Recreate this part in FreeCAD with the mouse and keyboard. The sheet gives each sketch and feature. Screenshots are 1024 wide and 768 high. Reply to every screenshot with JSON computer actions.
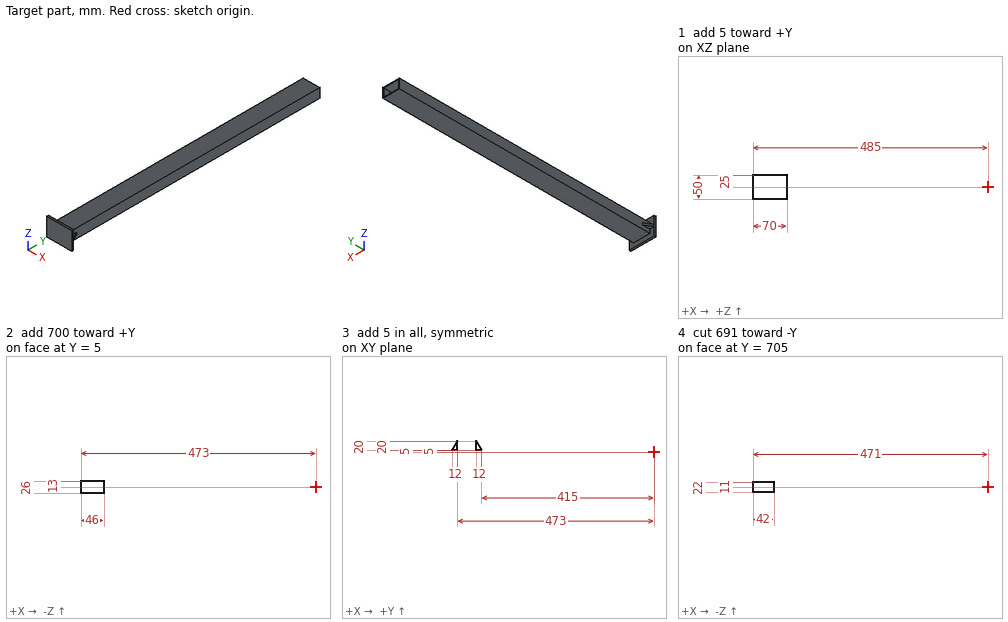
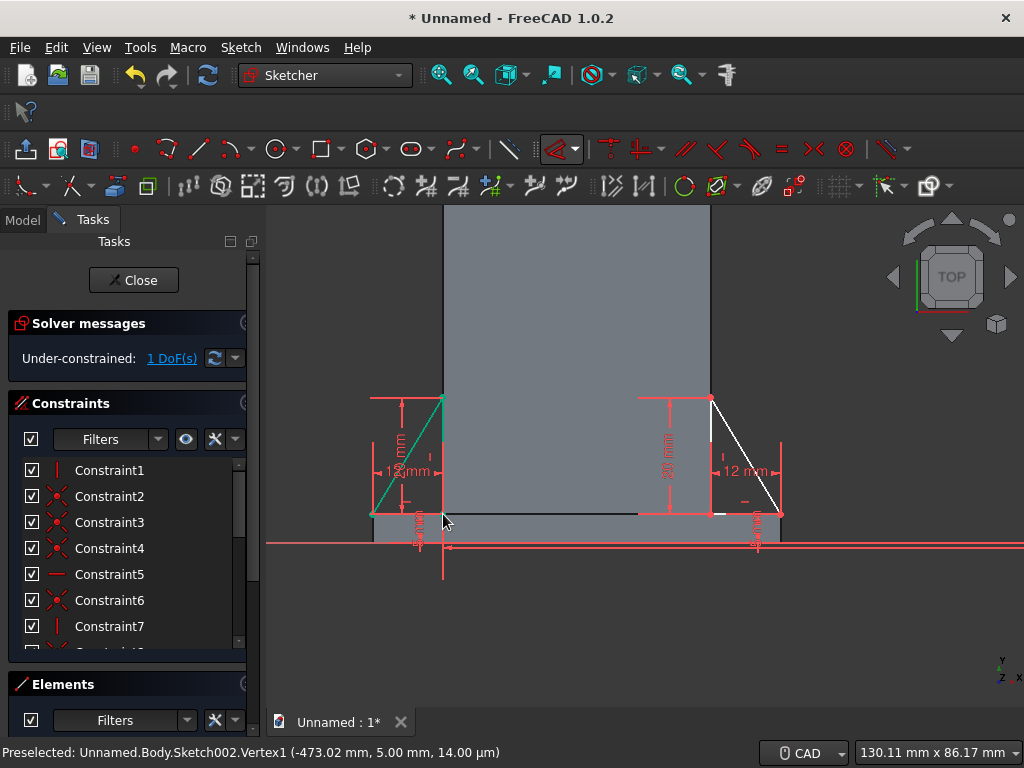
{"action": "left_click", "coordinate": [781, 514]}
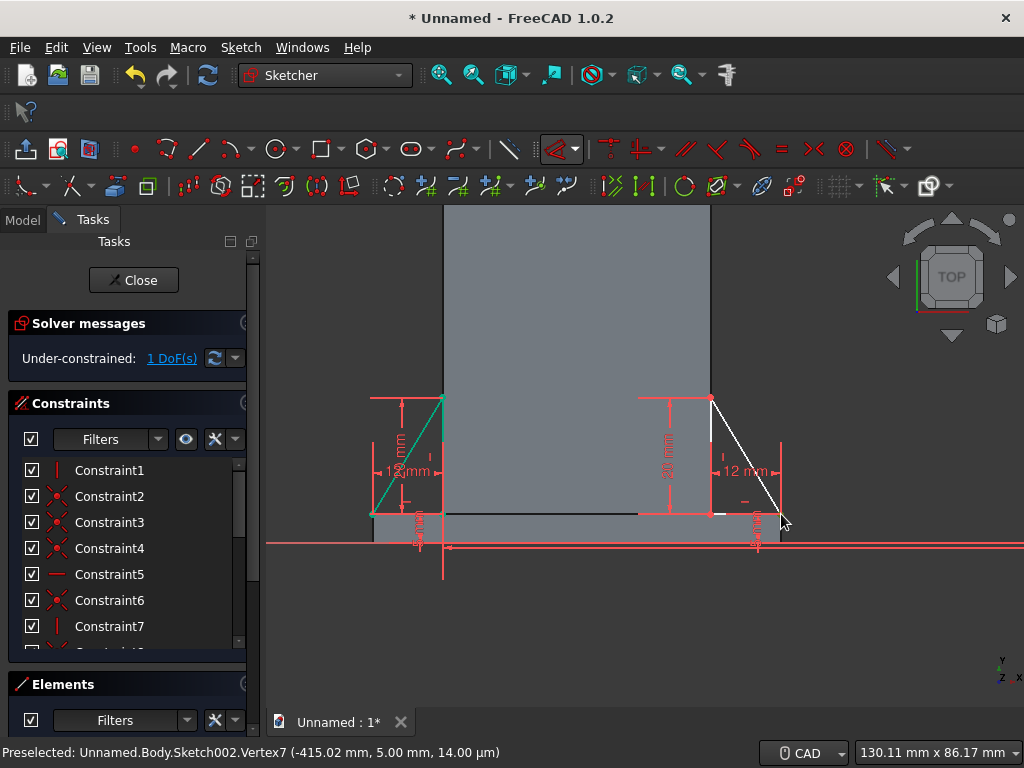
{"action": "left_click", "coordinate": [578, 150]}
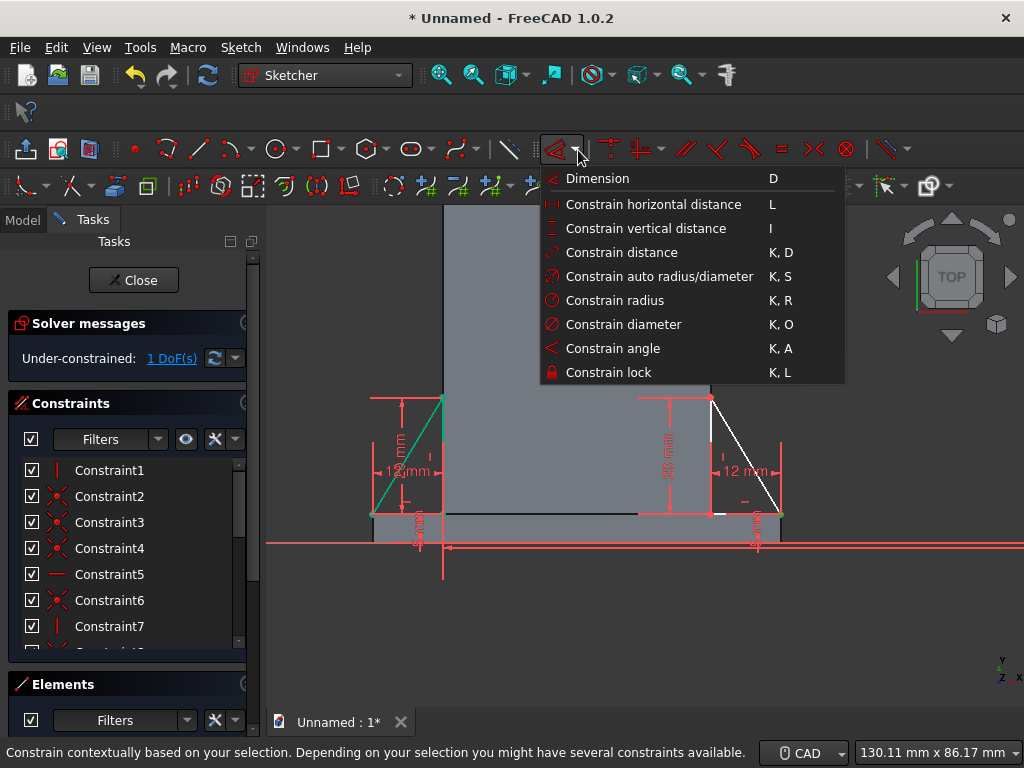
{"action": "left_click", "coordinate": [693, 204]}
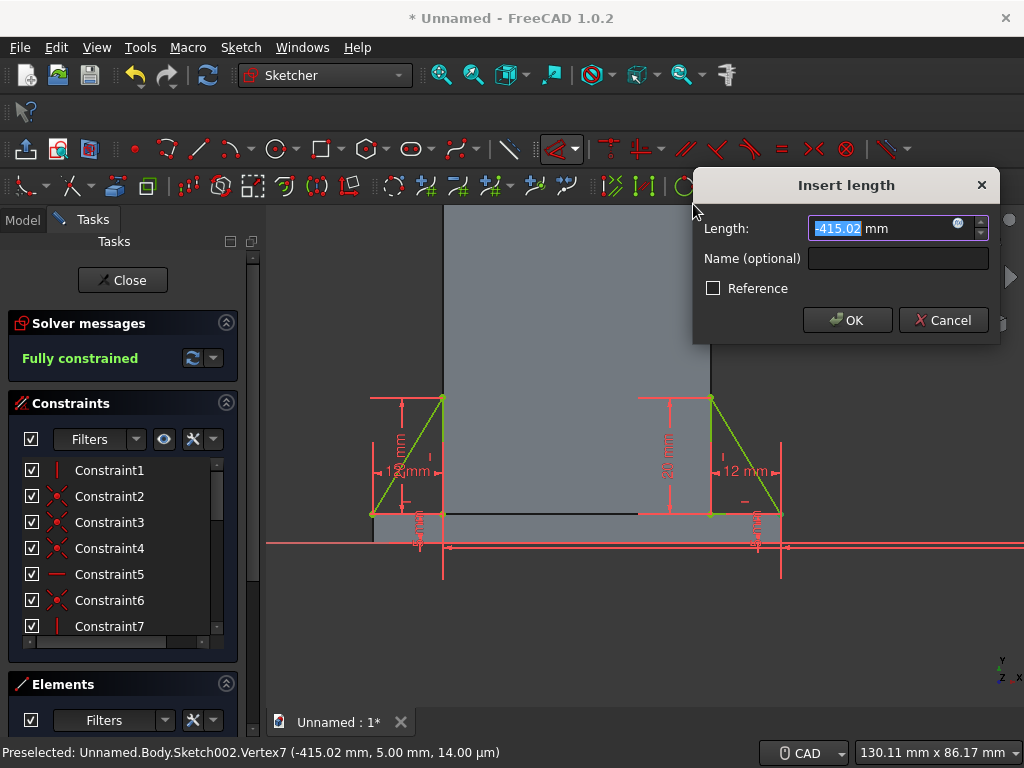
{"action": "type", "text": "-415"}
{"action": "key", "text": "Return"}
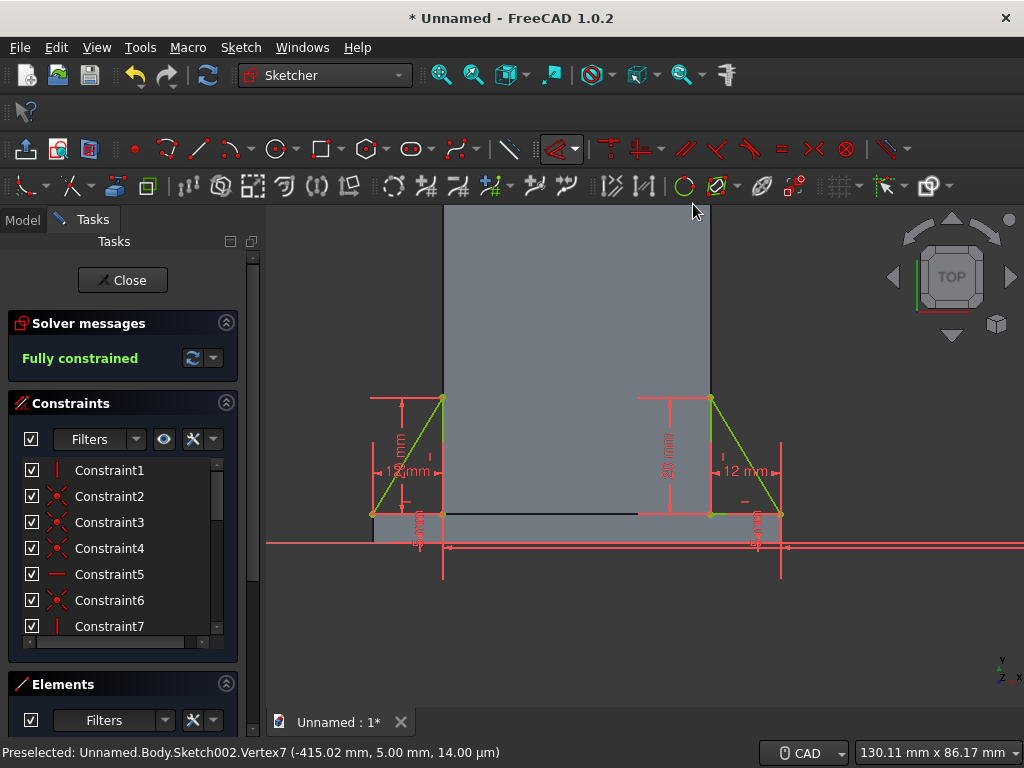
{"action": "left_click", "coordinate": [123, 280]}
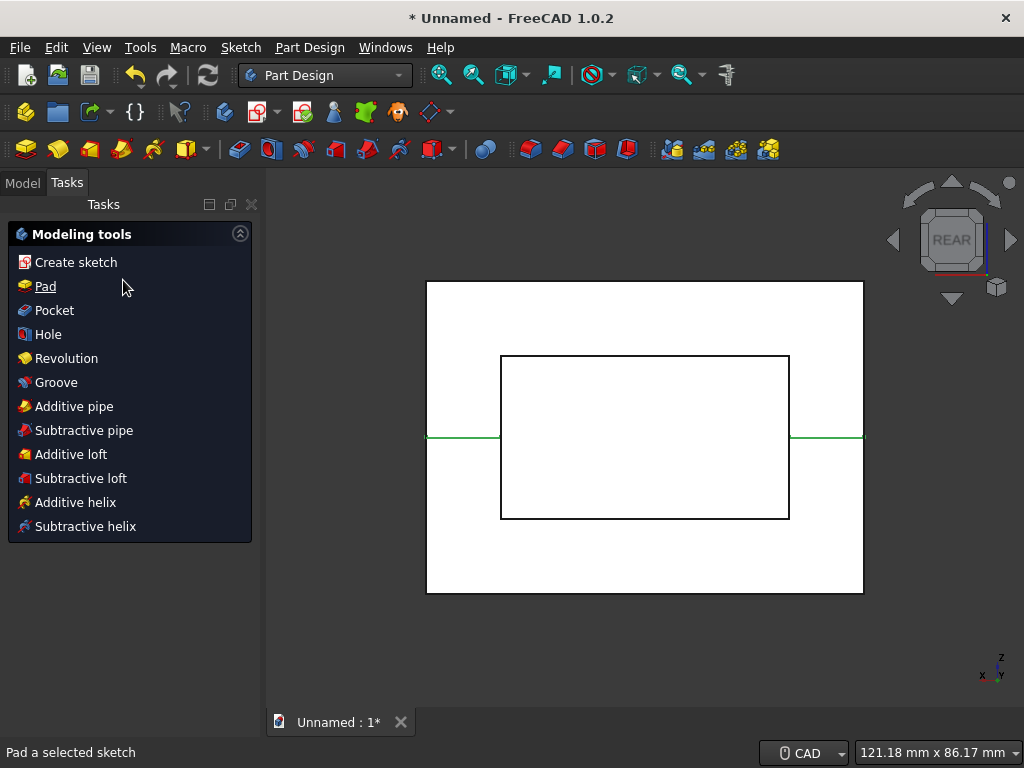
{"action": "left_click", "coordinate": [26, 150]}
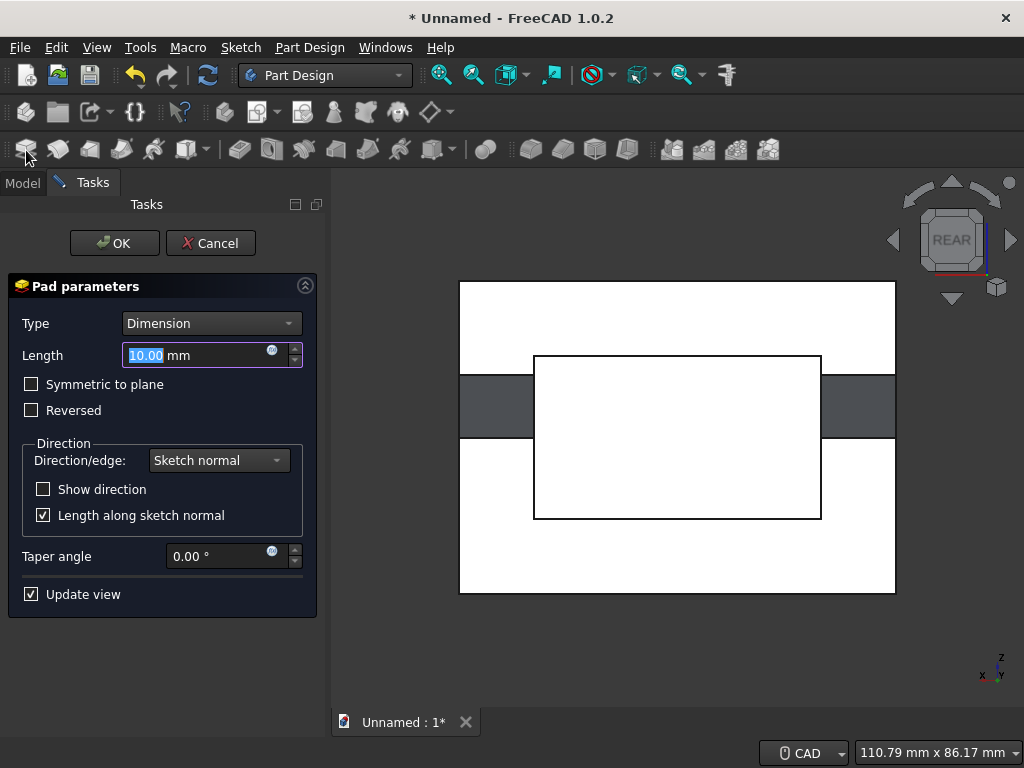
{"action": "type", "text": "5"}
{"action": "key", "text": "Tab"}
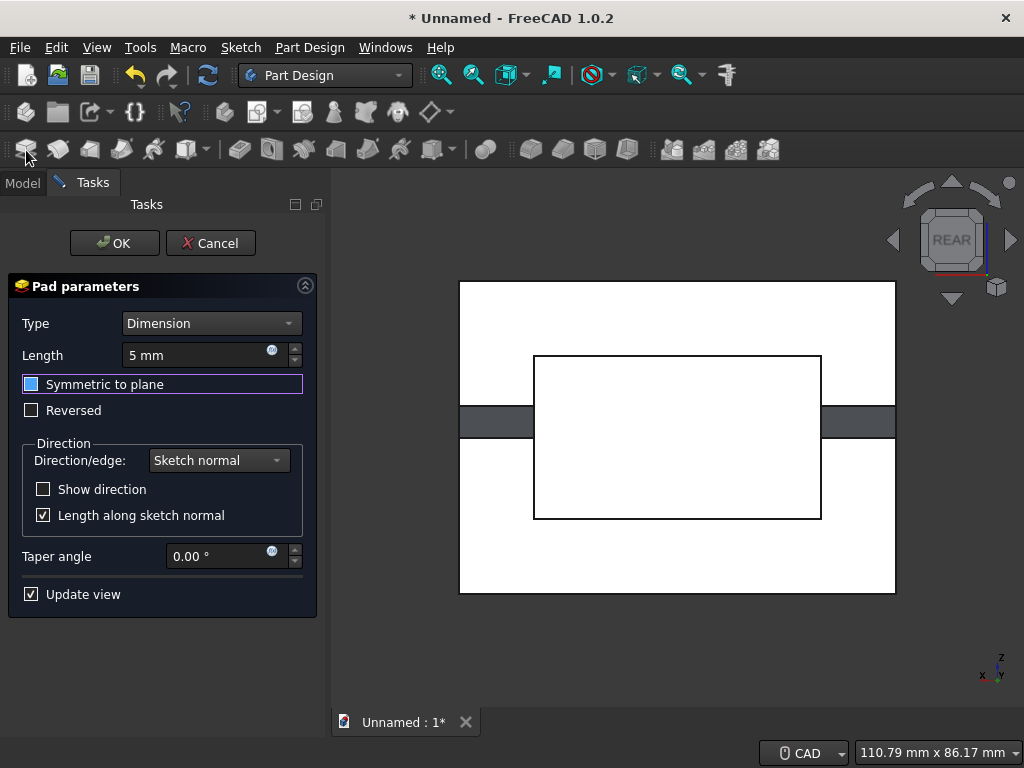
{"action": "left_click", "coordinate": [30, 384]}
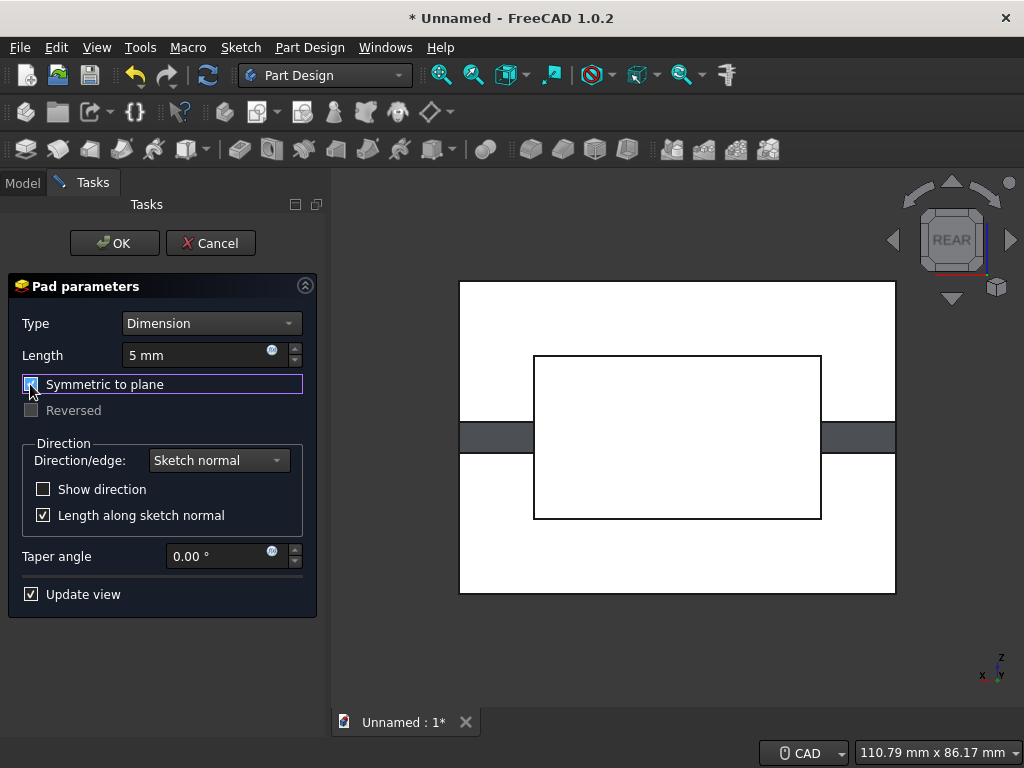
{"action": "left_click", "coordinate": [115, 243]}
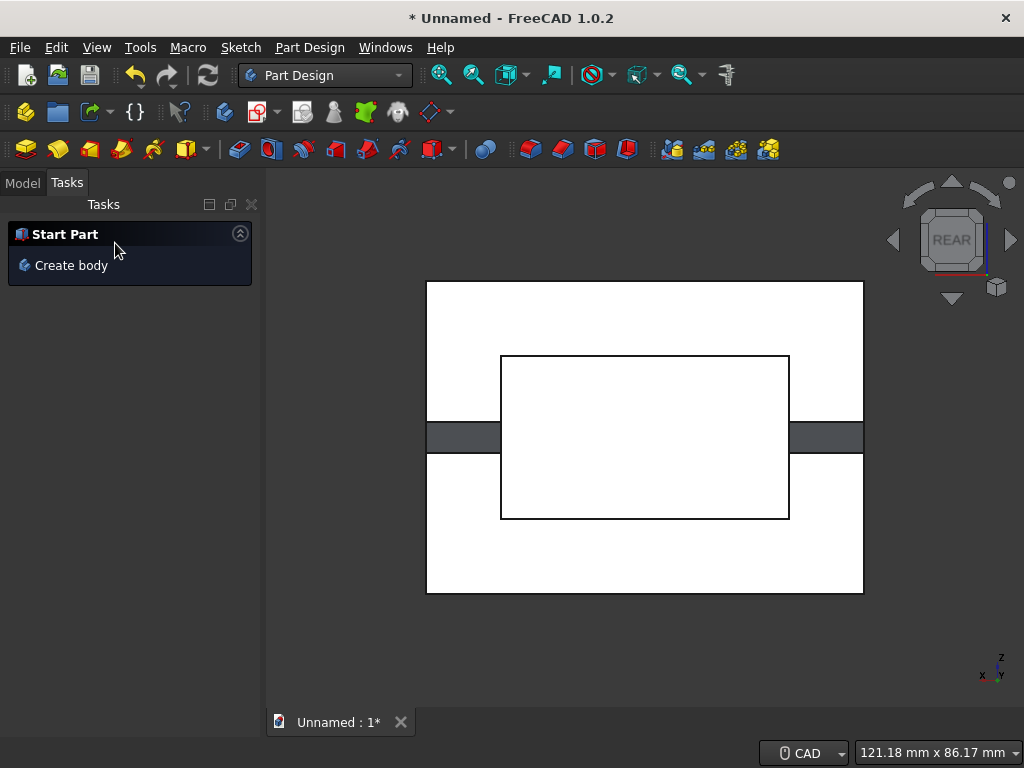
{"action": "left_click", "coordinate": [604, 436]}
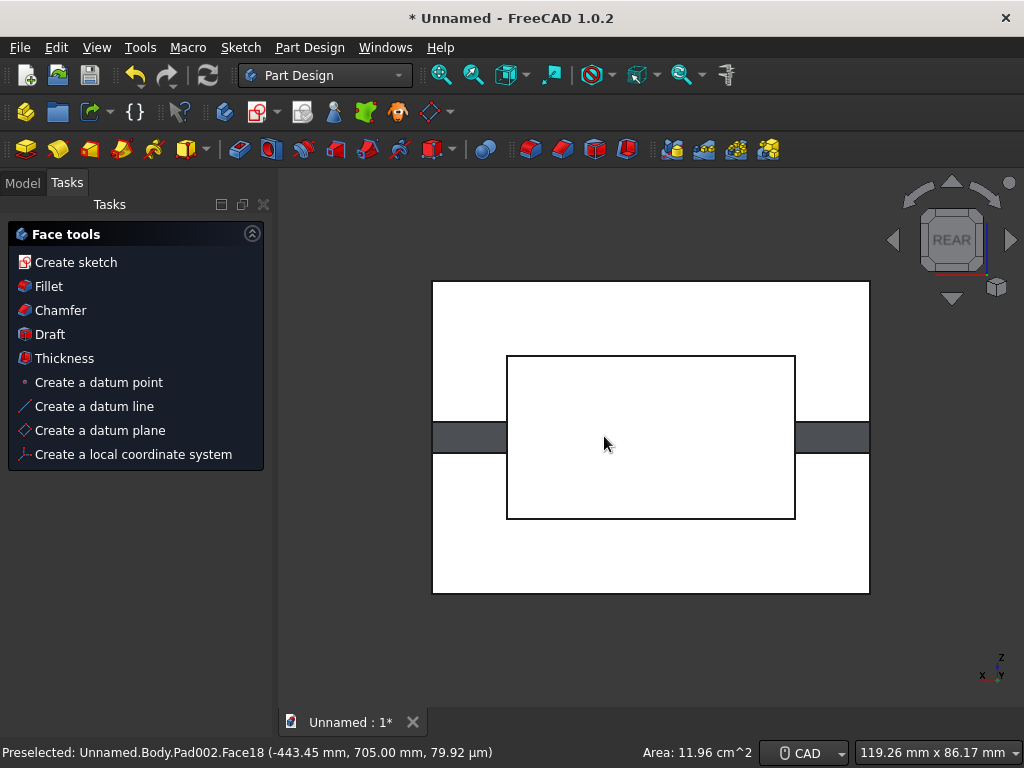
{"action": "left_click", "coordinate": [258, 112]}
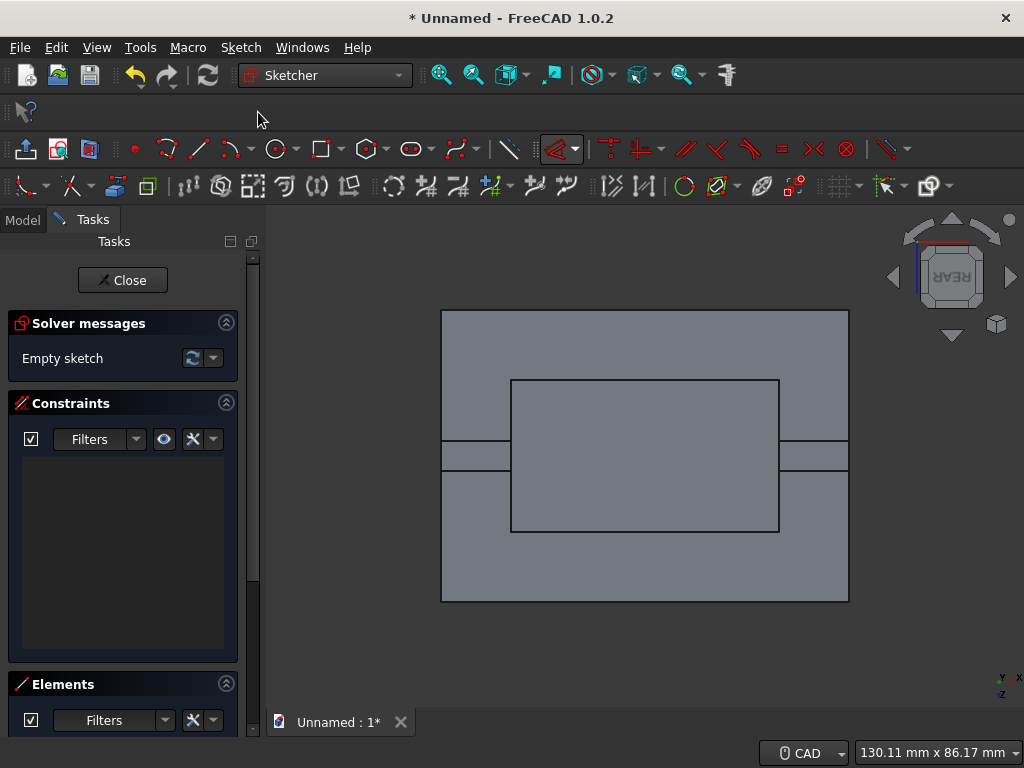
{"action": "scroll", "coordinate": [784, 456], "scroll_direction": "up", "scroll_amount": 2}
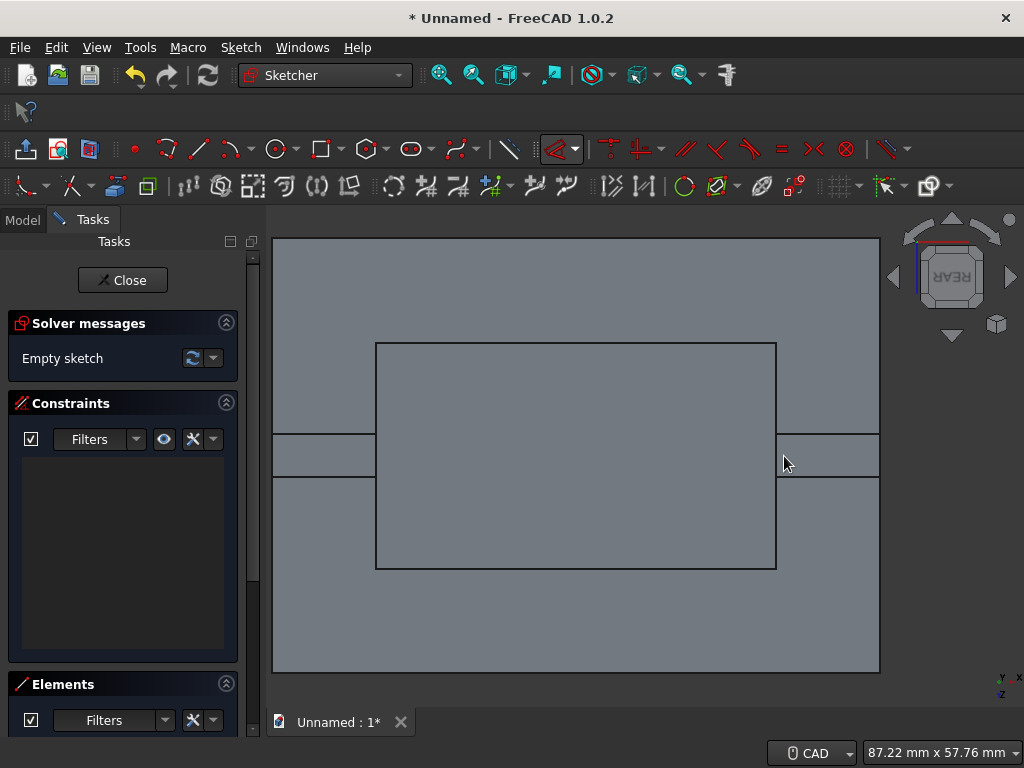
{"action": "left_click", "coordinate": [322, 150]}